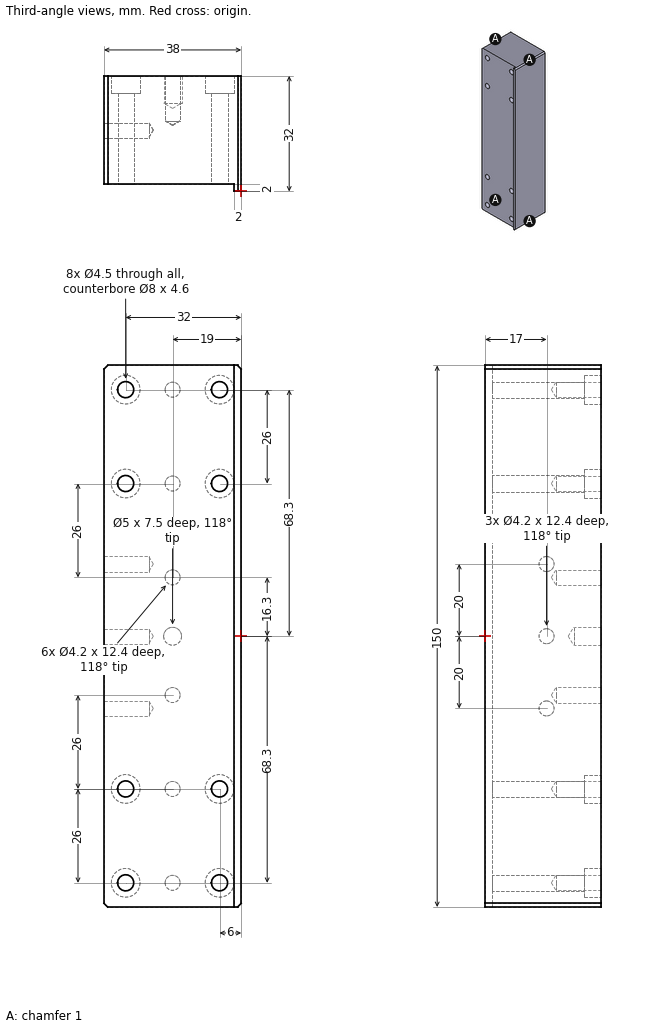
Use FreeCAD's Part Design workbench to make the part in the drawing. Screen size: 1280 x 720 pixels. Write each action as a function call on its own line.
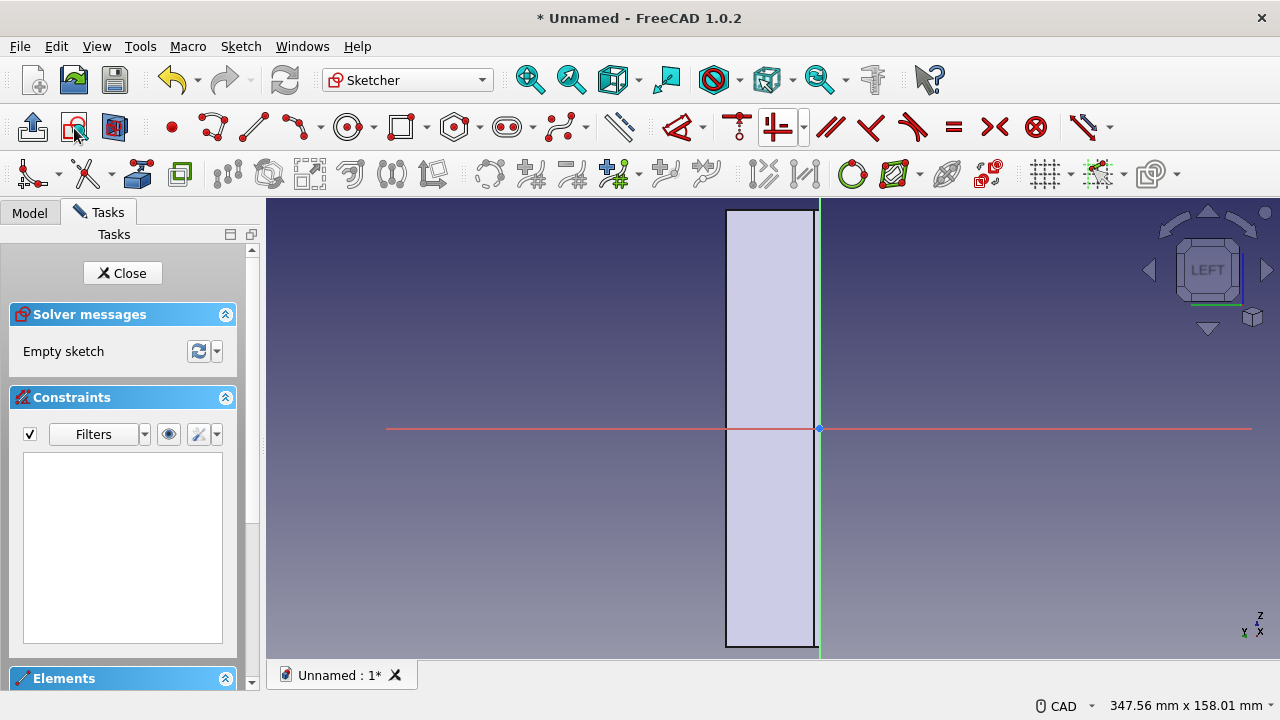
scroll(863, 429, up, 4)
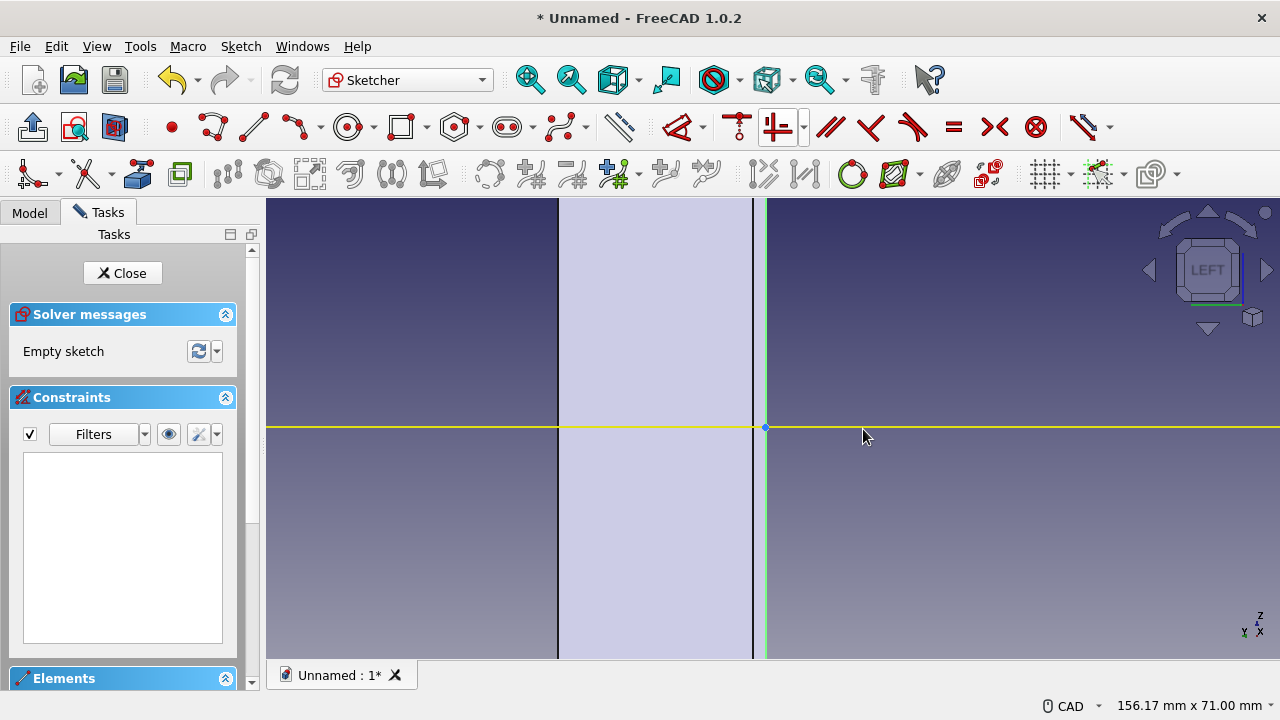
click(348, 128)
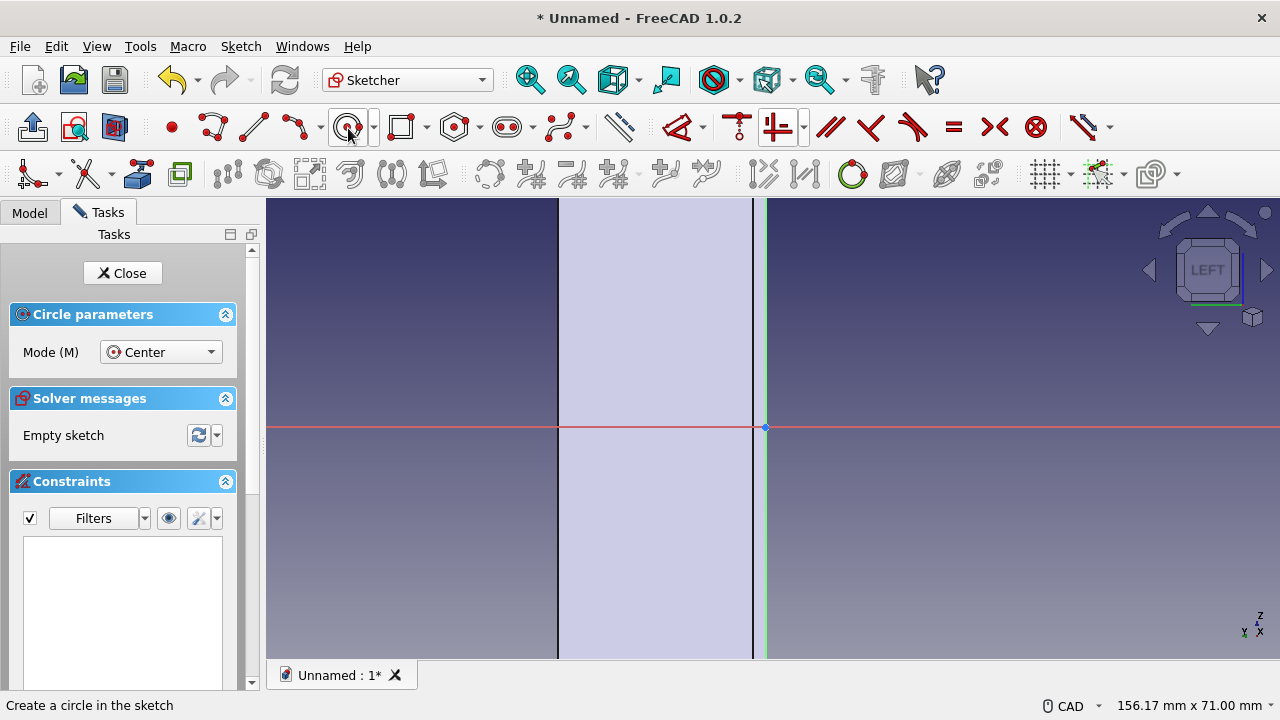
scroll(655, 427, up, 3)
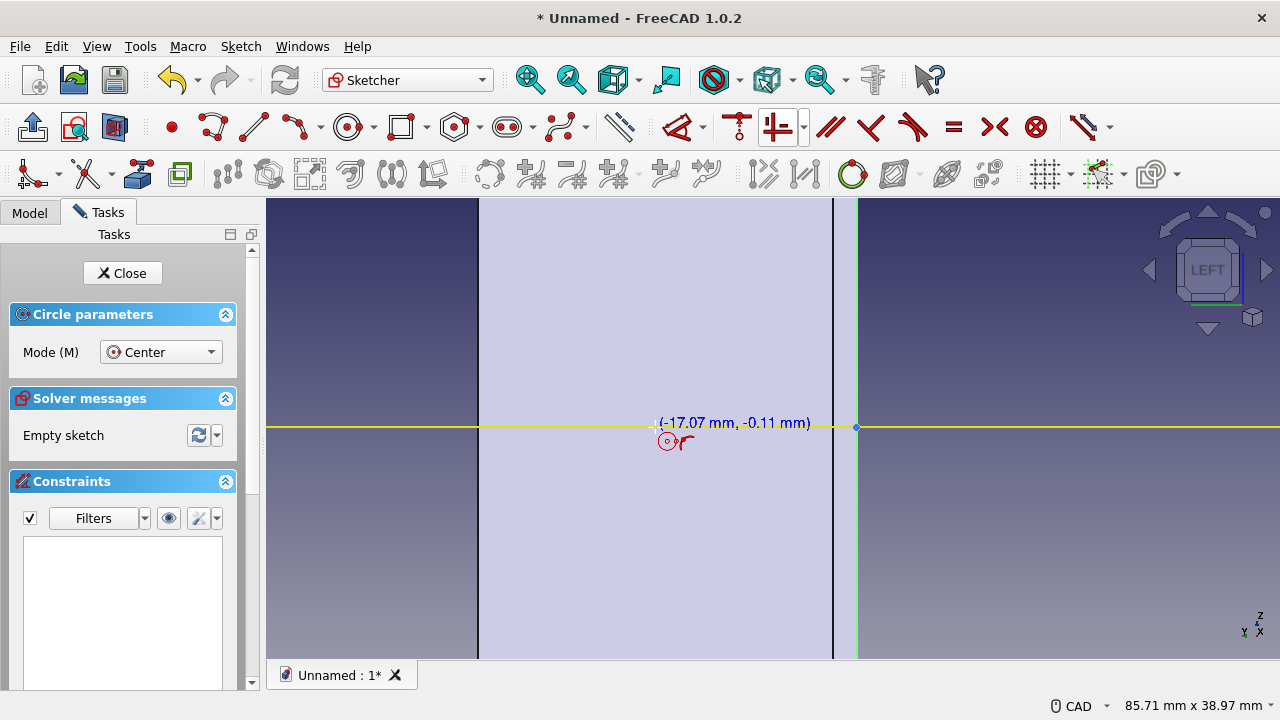
click(656, 427)
move(673, 410)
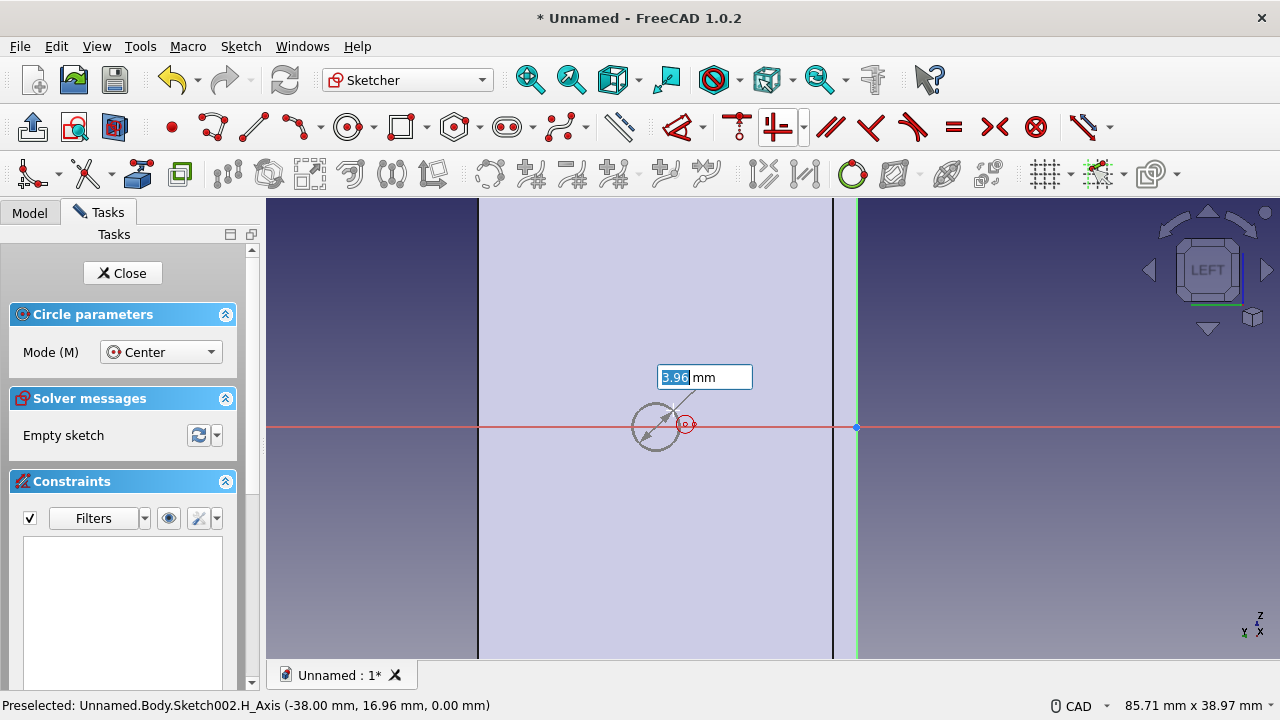
text(4.2)
key(Return)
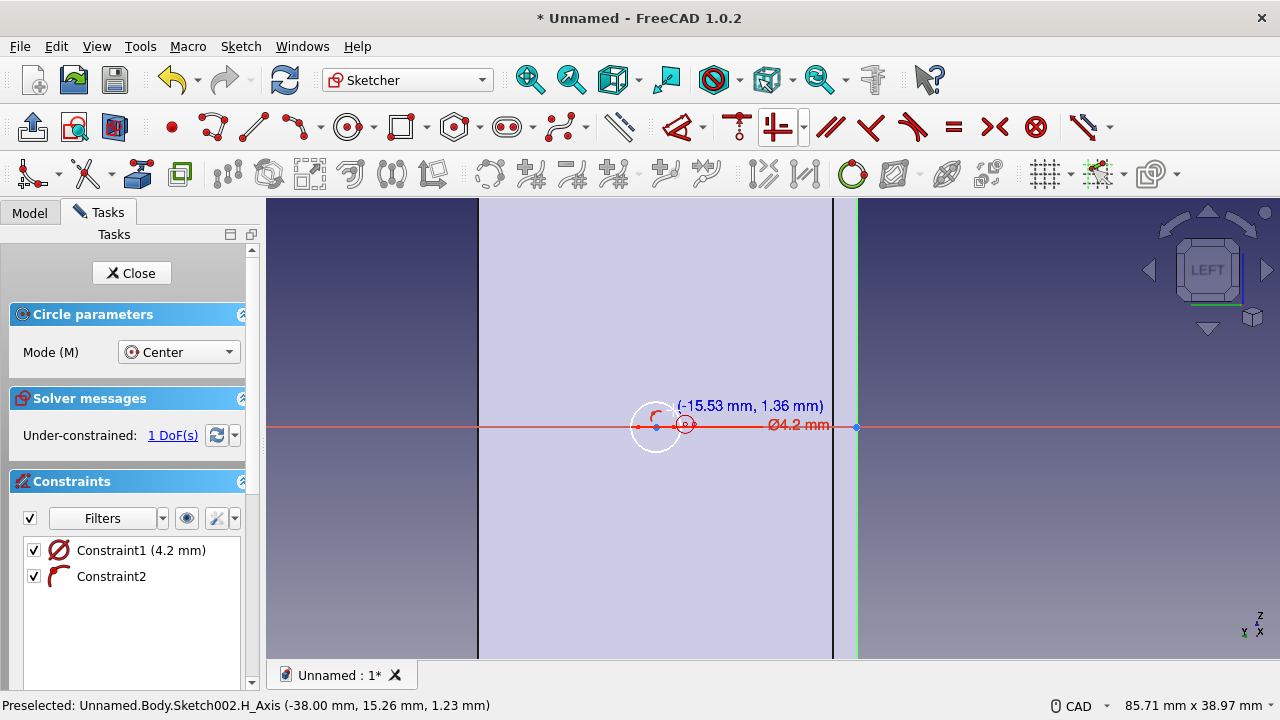
scroll(657, 430, down, 3)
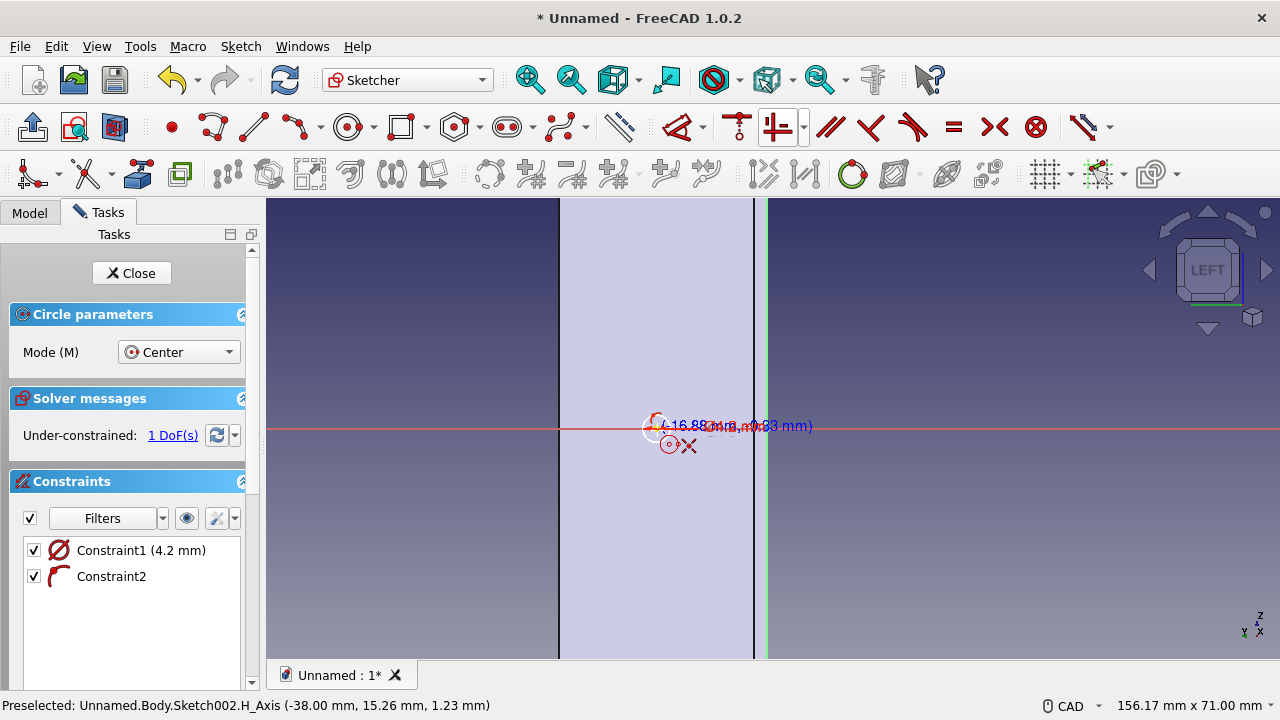
scroll(656, 299, up, 3)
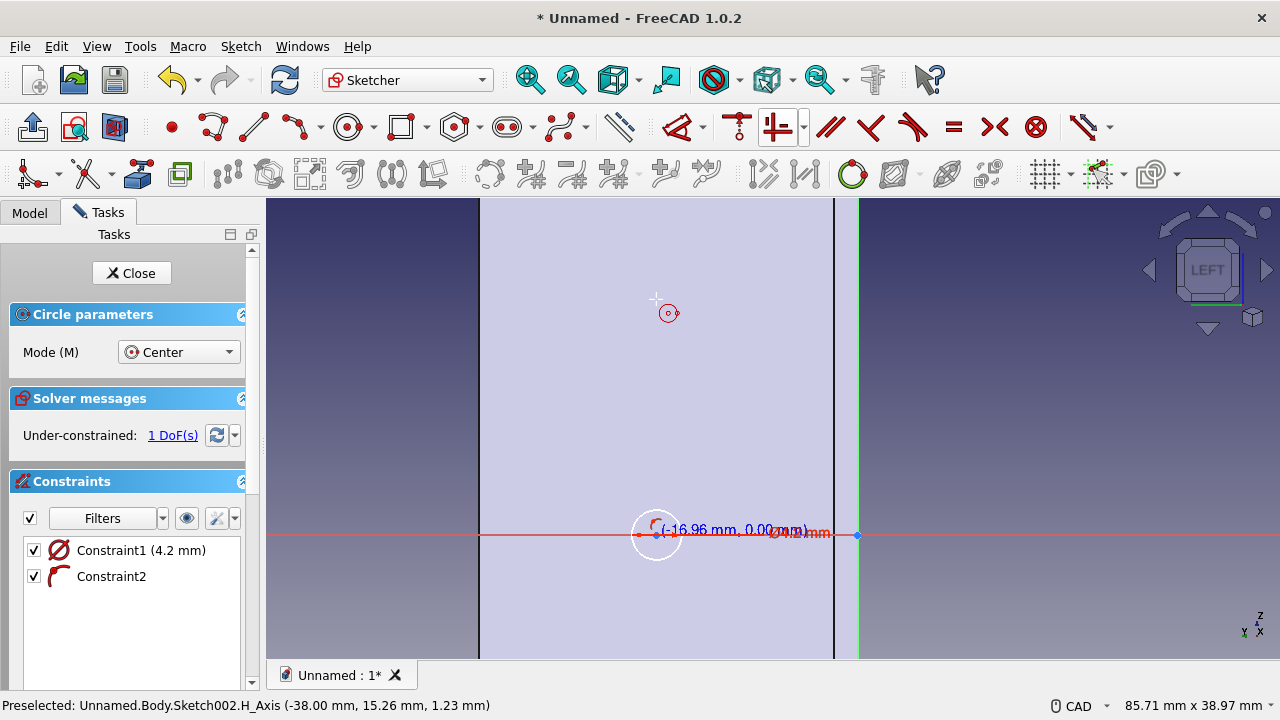
click(656, 298)
move(674, 281)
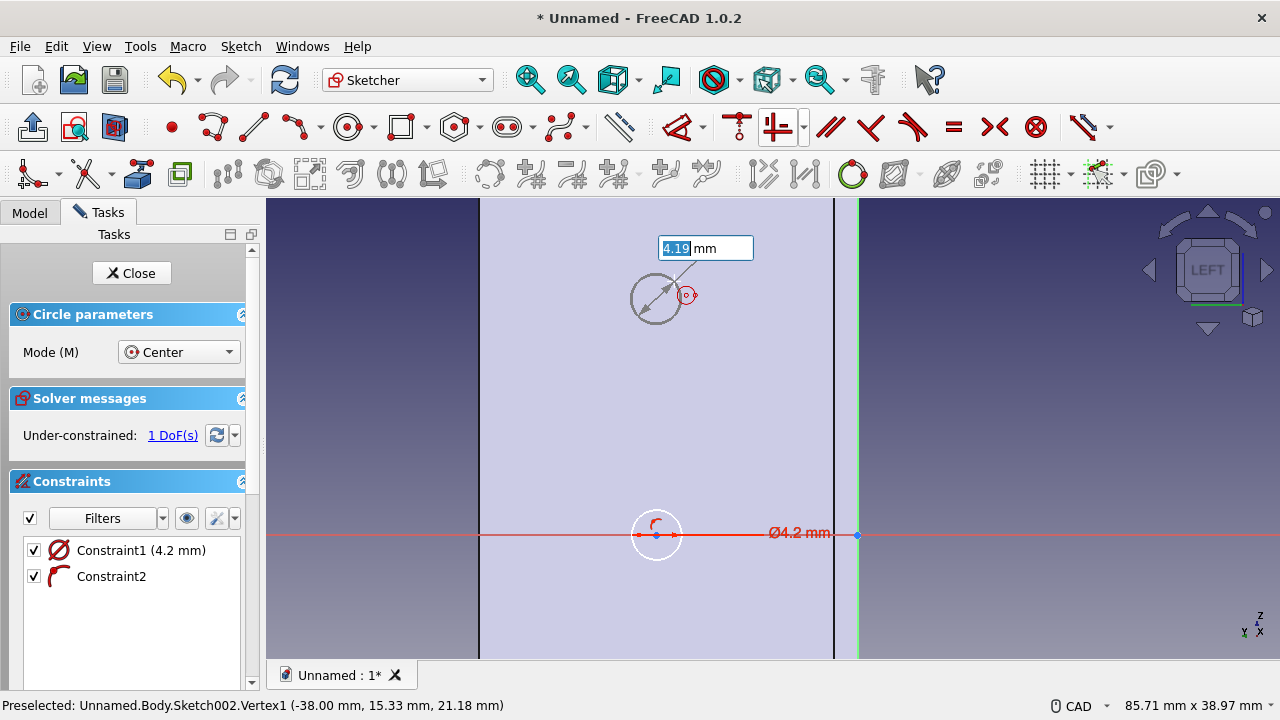
text(4.2)
key(Return)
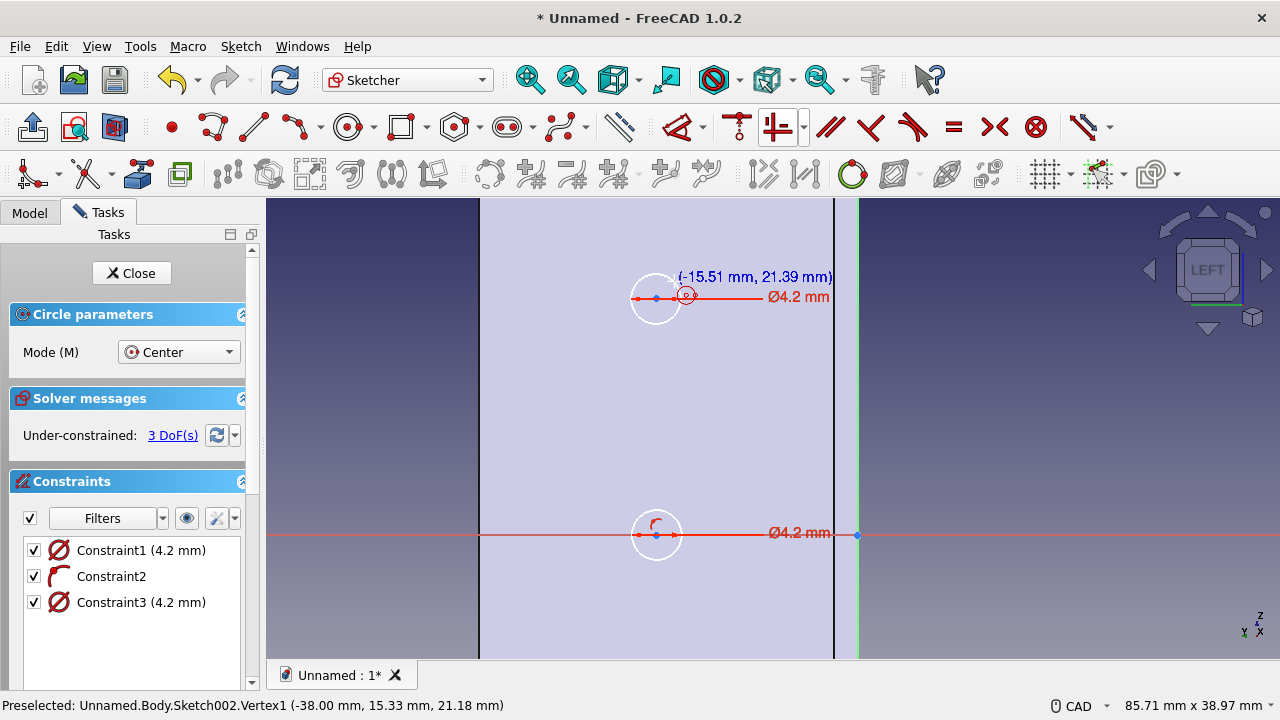
scroll(656, 299, down, 3)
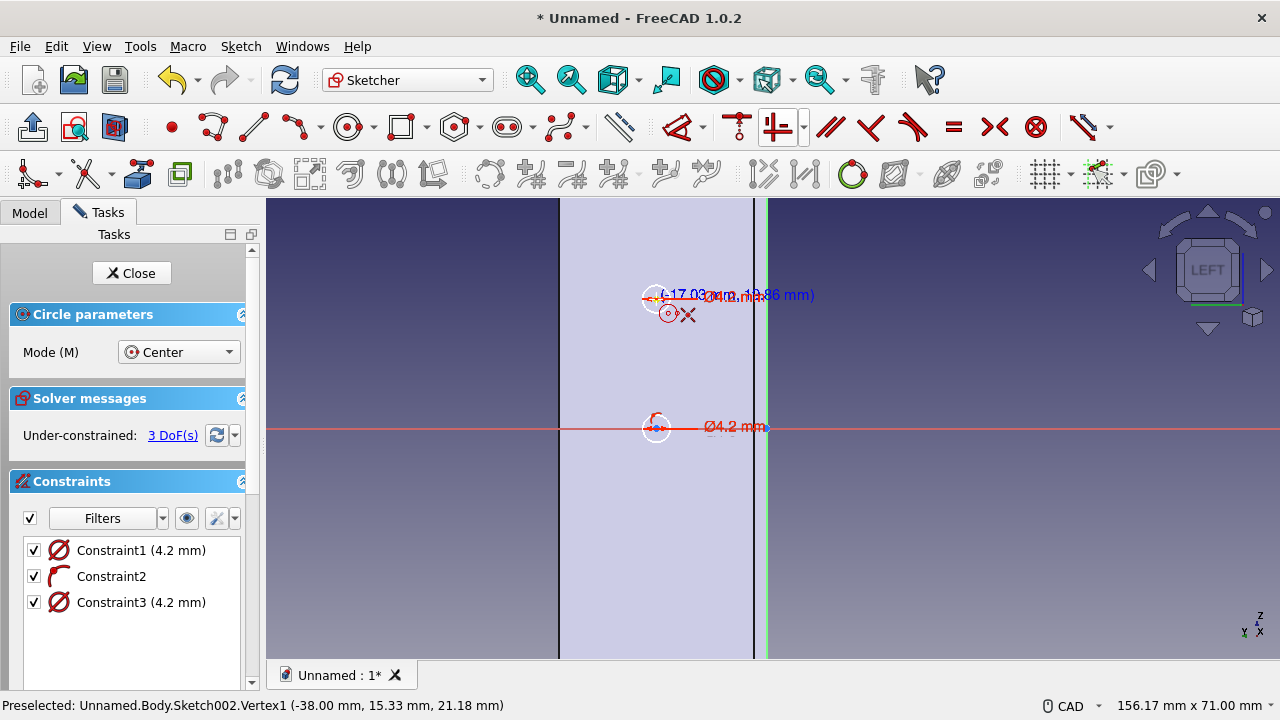
scroll(656, 558, up, 3)